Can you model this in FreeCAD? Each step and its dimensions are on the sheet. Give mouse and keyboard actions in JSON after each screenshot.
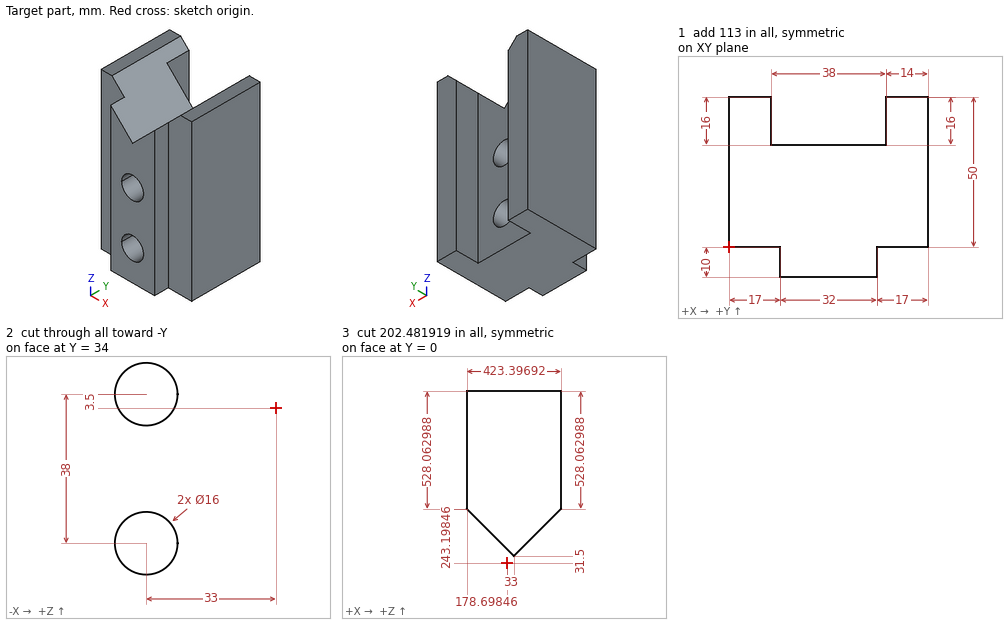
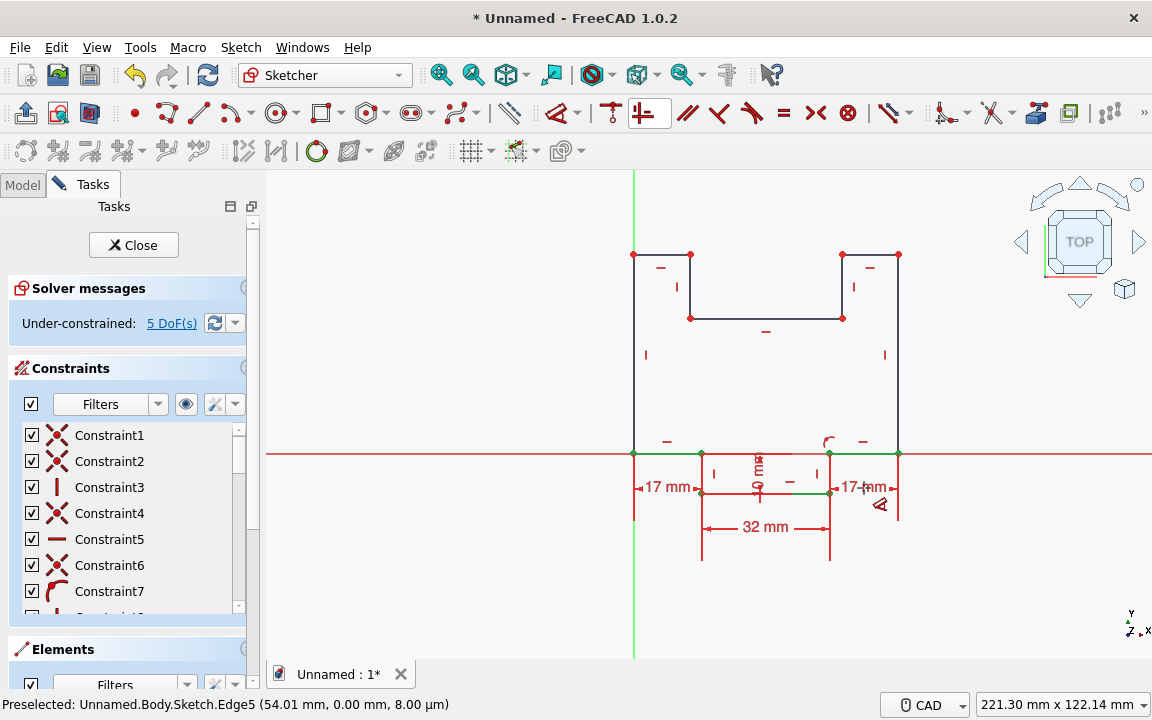
{"action": "left_click", "coordinate": [898, 394]}
{"action": "left_click", "coordinate": [932, 354]}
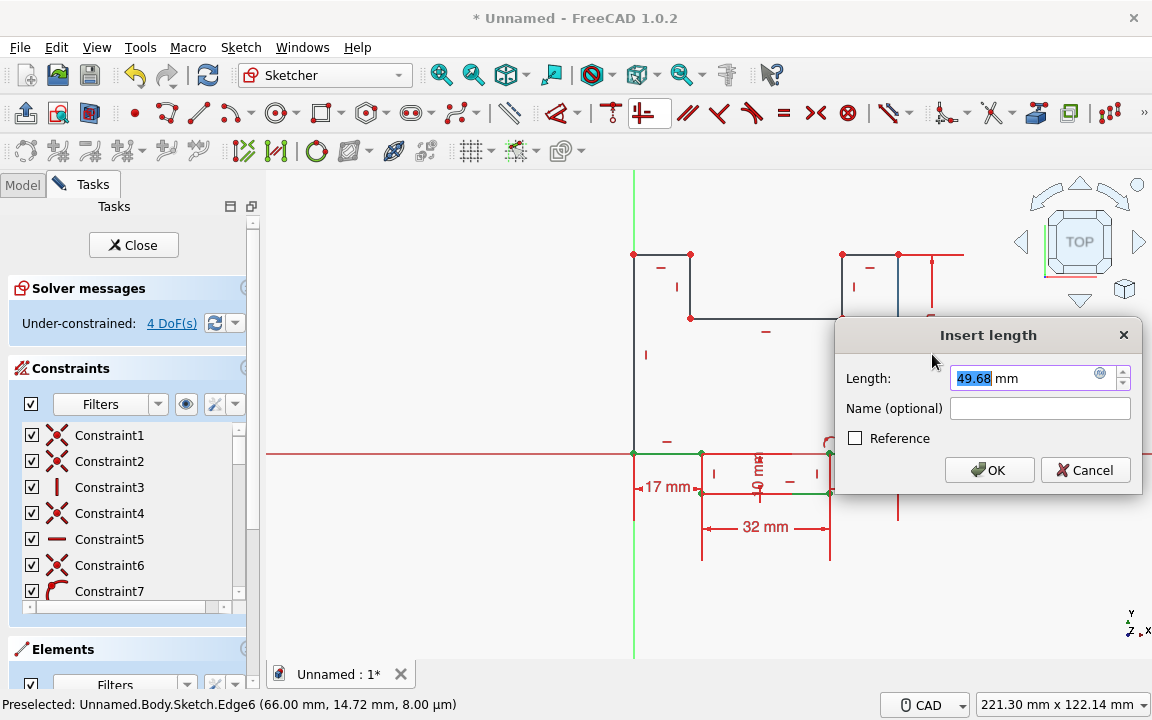
{"action": "type", "text": "50"}
{"action": "key", "text": "Return"}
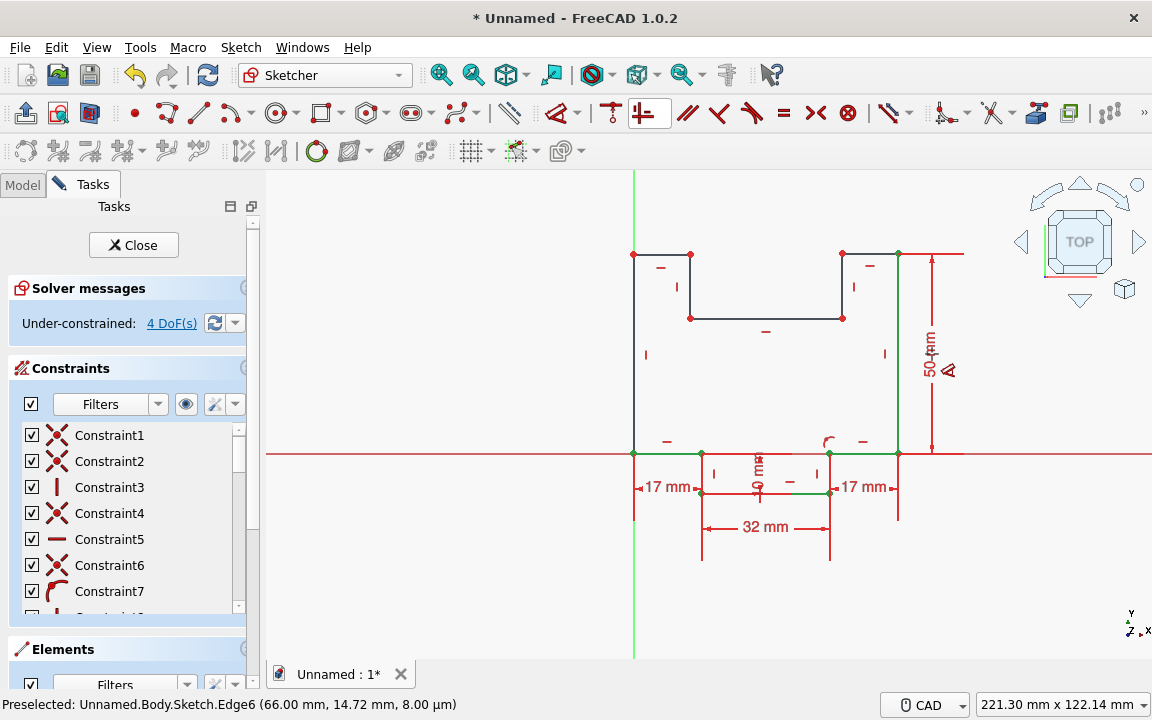
{"action": "left_click", "coordinate": [881, 254]}
{"action": "left_click", "coordinate": [870, 220]}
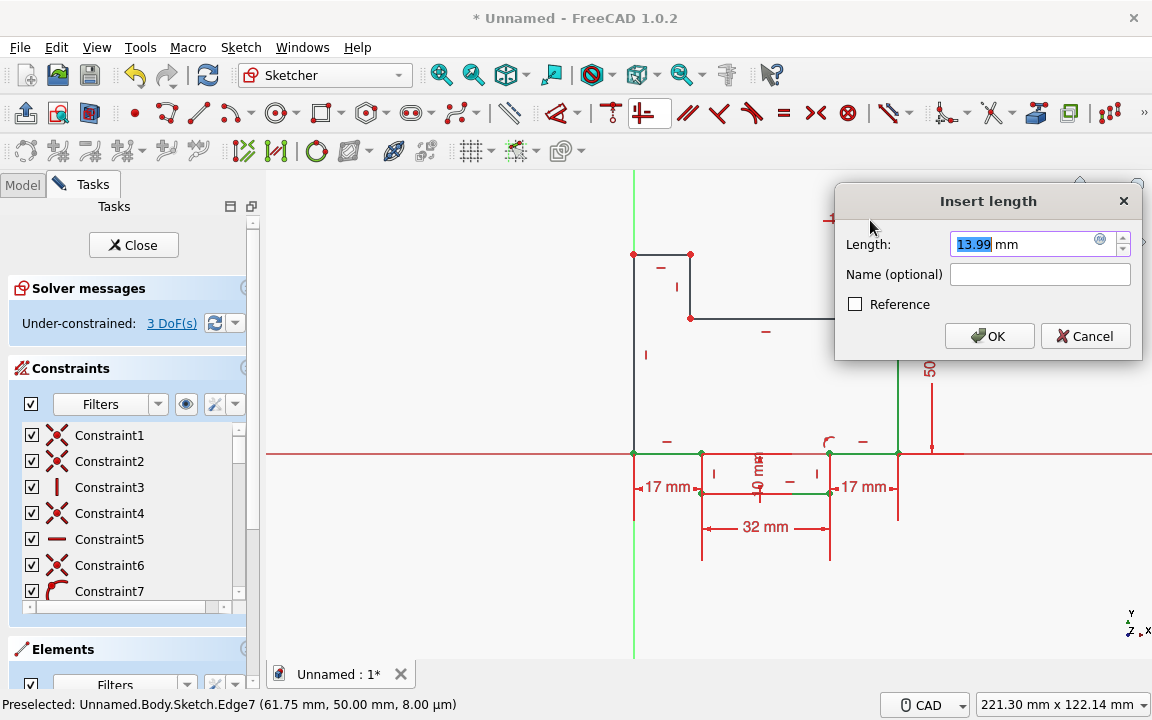
{"action": "type", "text": "14"}
{"action": "key", "text": "Return"}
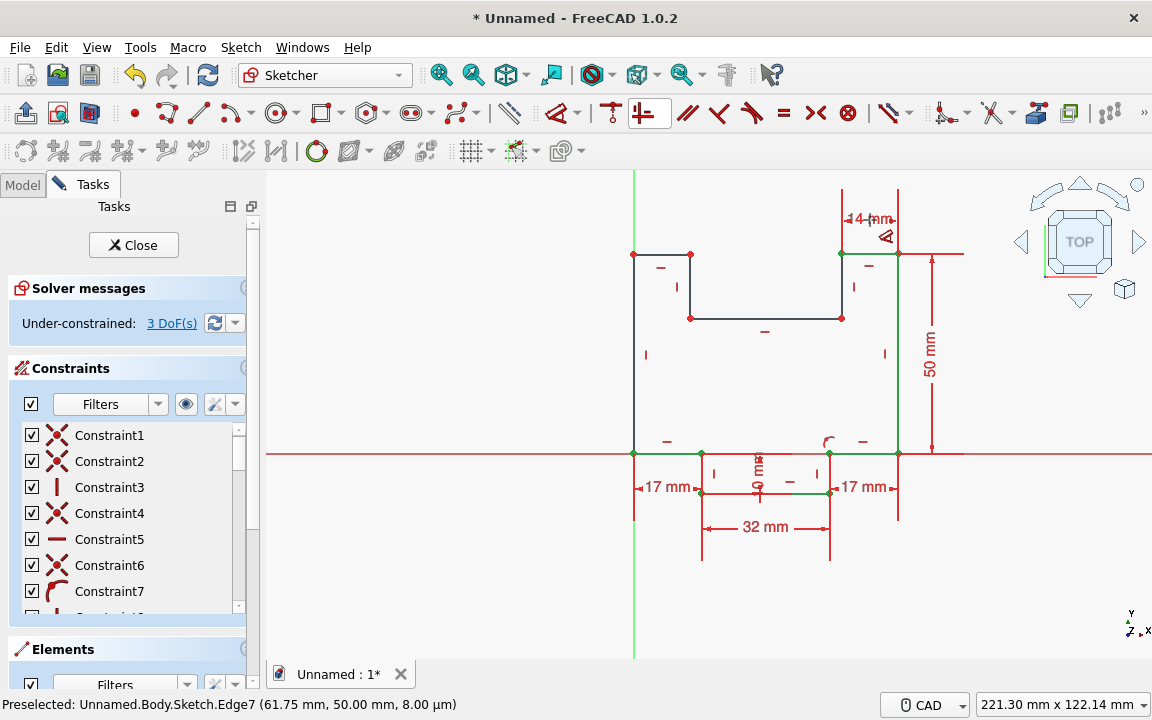
{"action": "left_click", "coordinate": [842, 273]}
{"action": "left_click", "coordinate": [876, 286]}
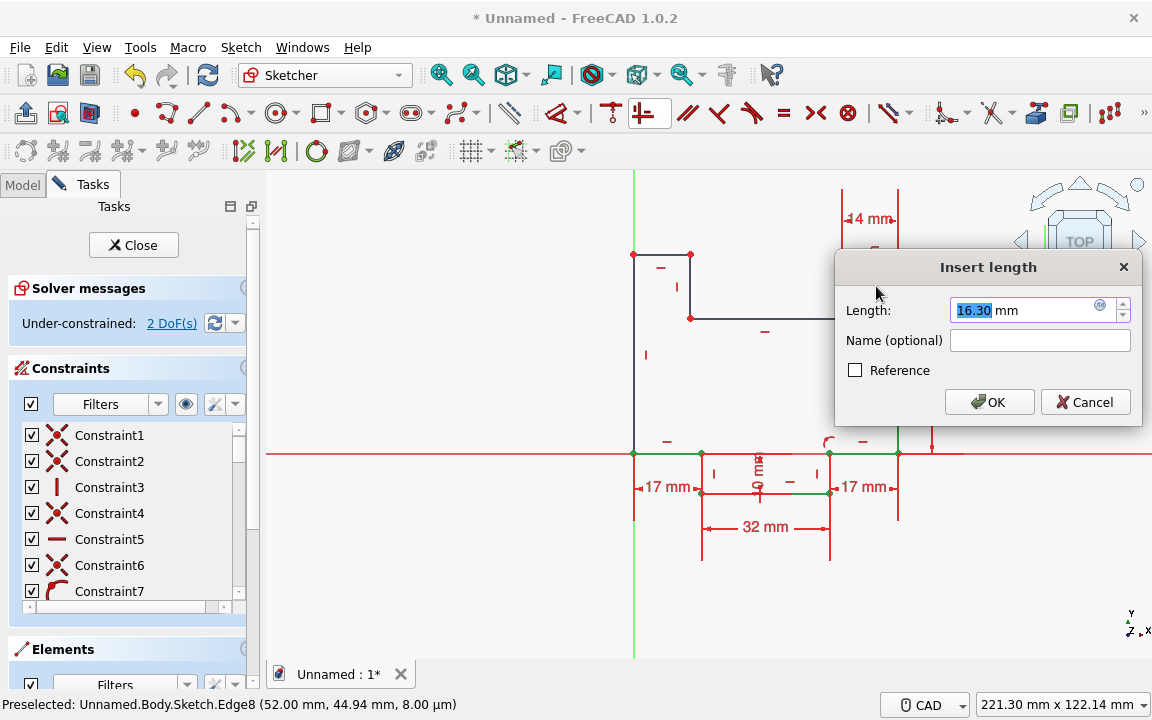
{"action": "type", "text": "16"}
{"action": "key", "text": "Return"}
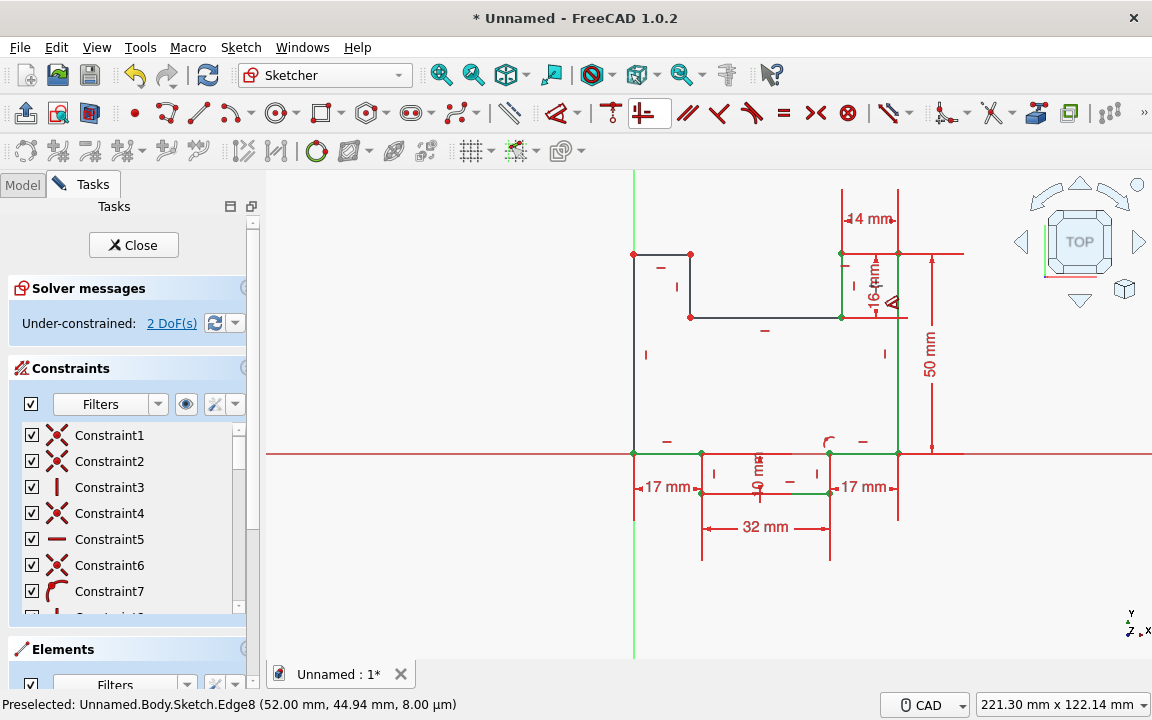
{"action": "left_click", "coordinate": [796, 318]}
{"action": "left_click", "coordinate": [766, 284]}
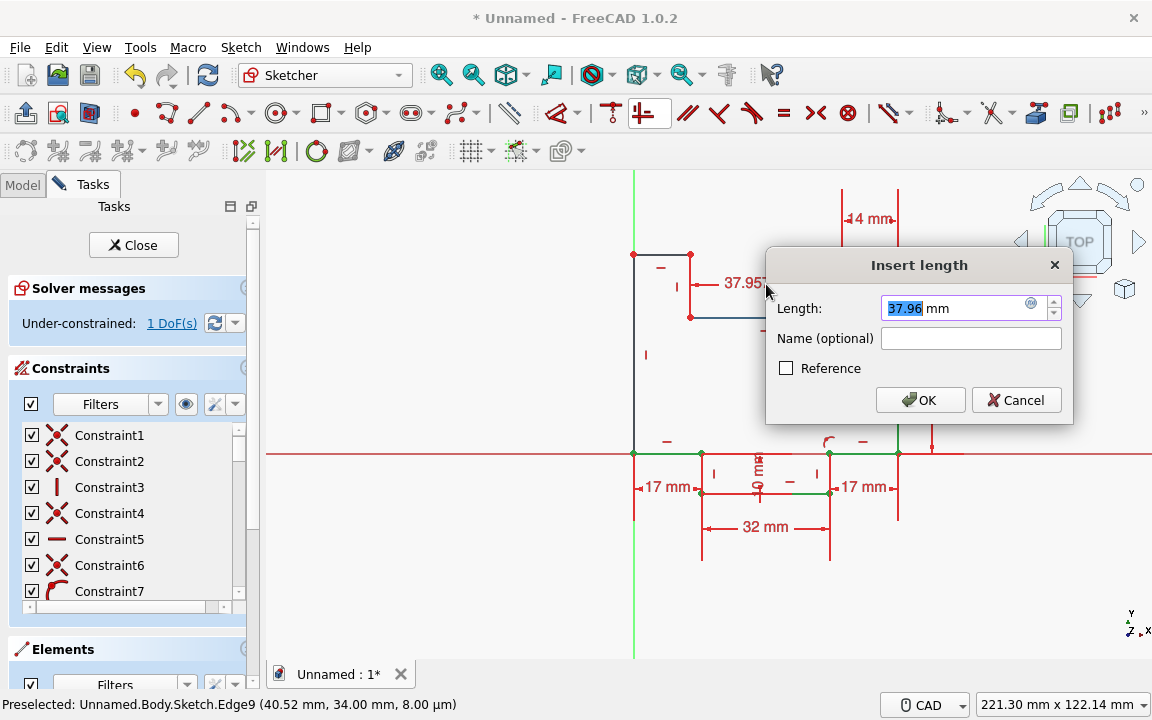
{"action": "type", "text": "38"}
{"action": "key", "text": "Return"}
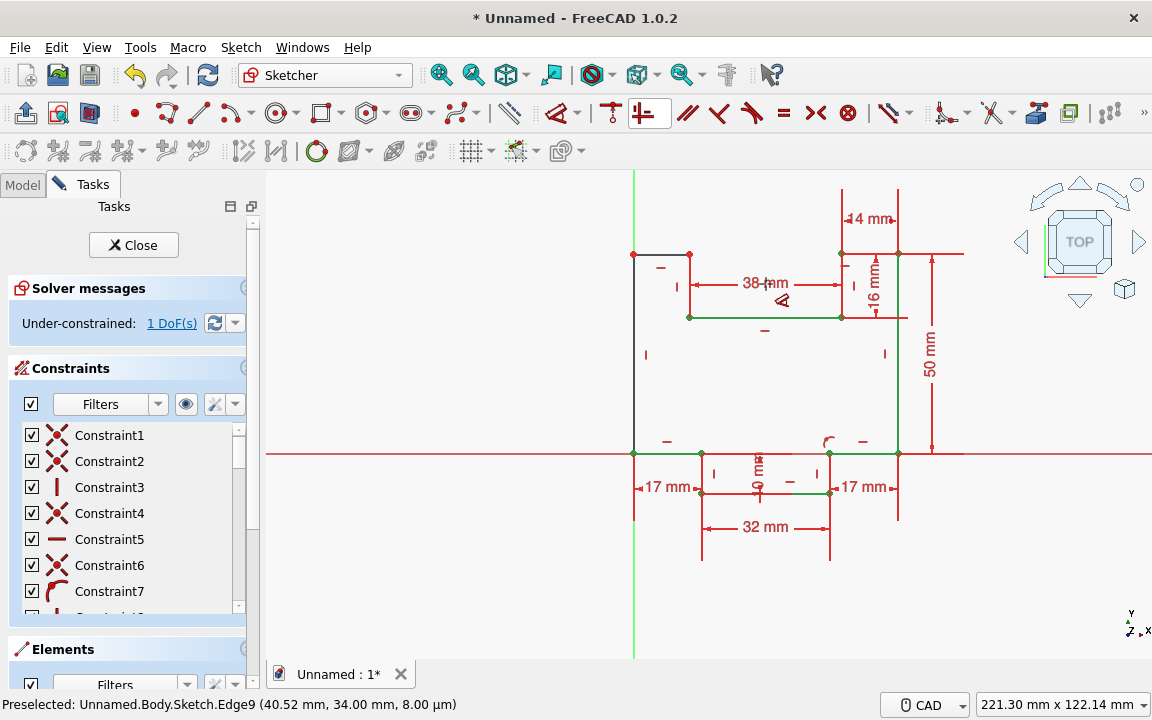
{"action": "left_click", "coordinate": [690, 299]}
{"action": "left_click", "coordinate": [656, 286]}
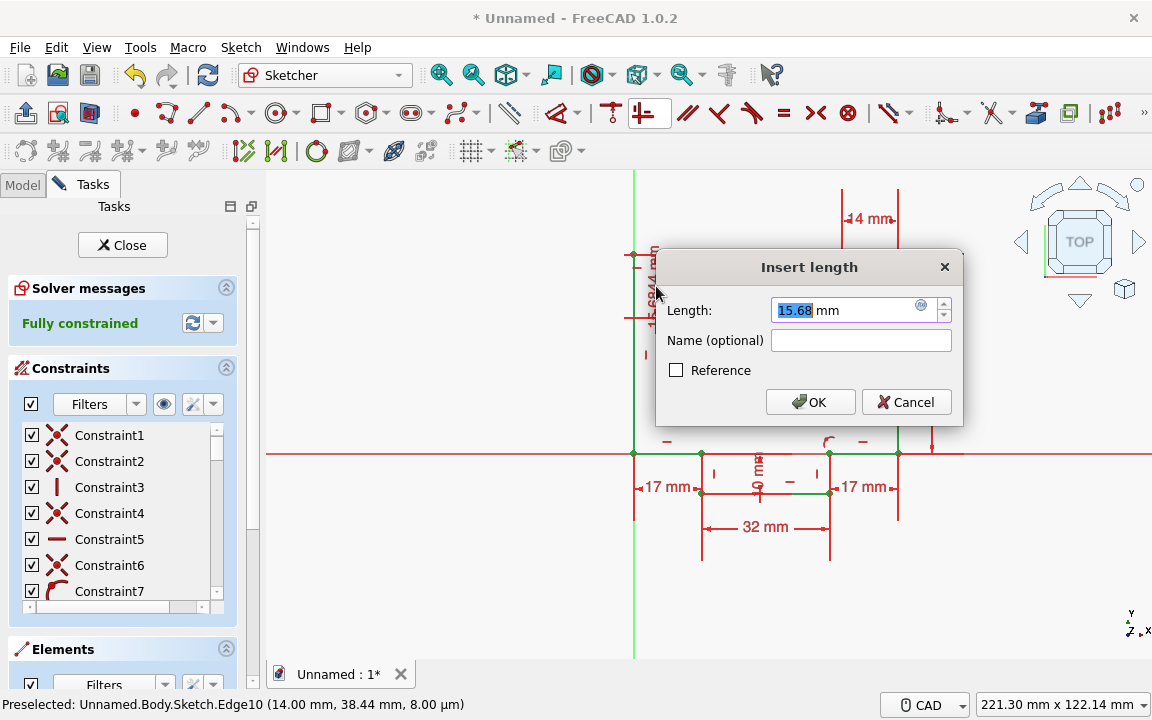
{"action": "type", "text": "16"}
{"action": "key", "text": "Return"}
{"action": "key", "text": "Escape"}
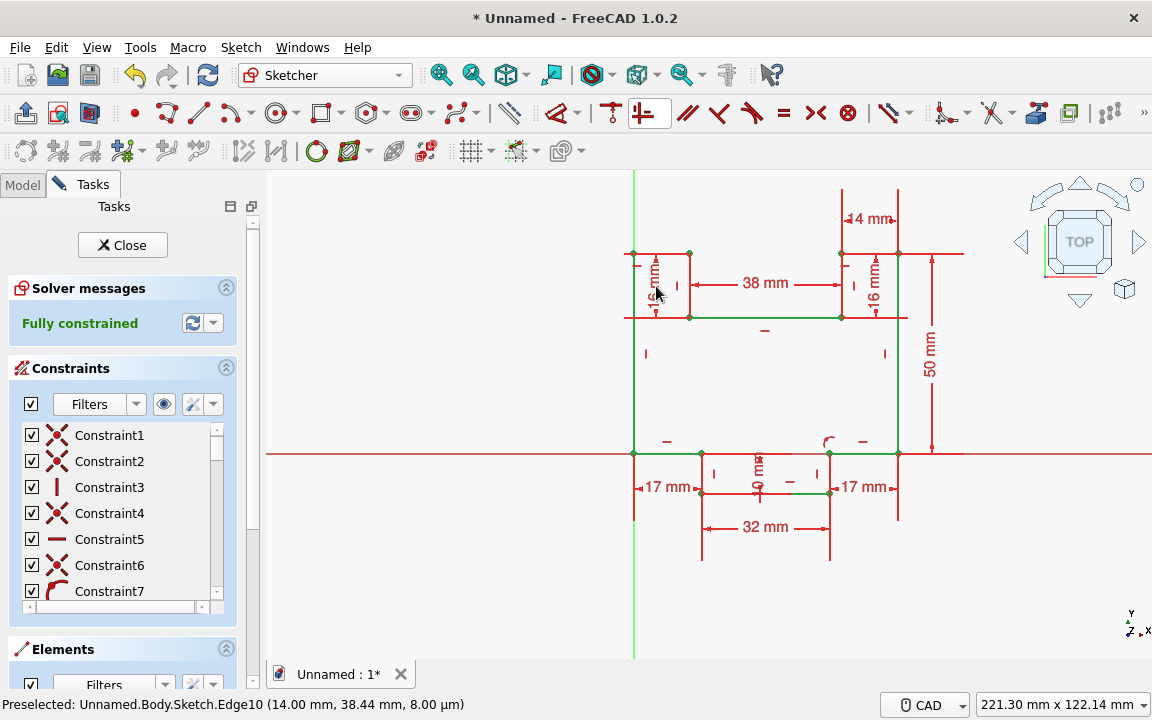
{"action": "left_click", "coordinate": [123, 245]}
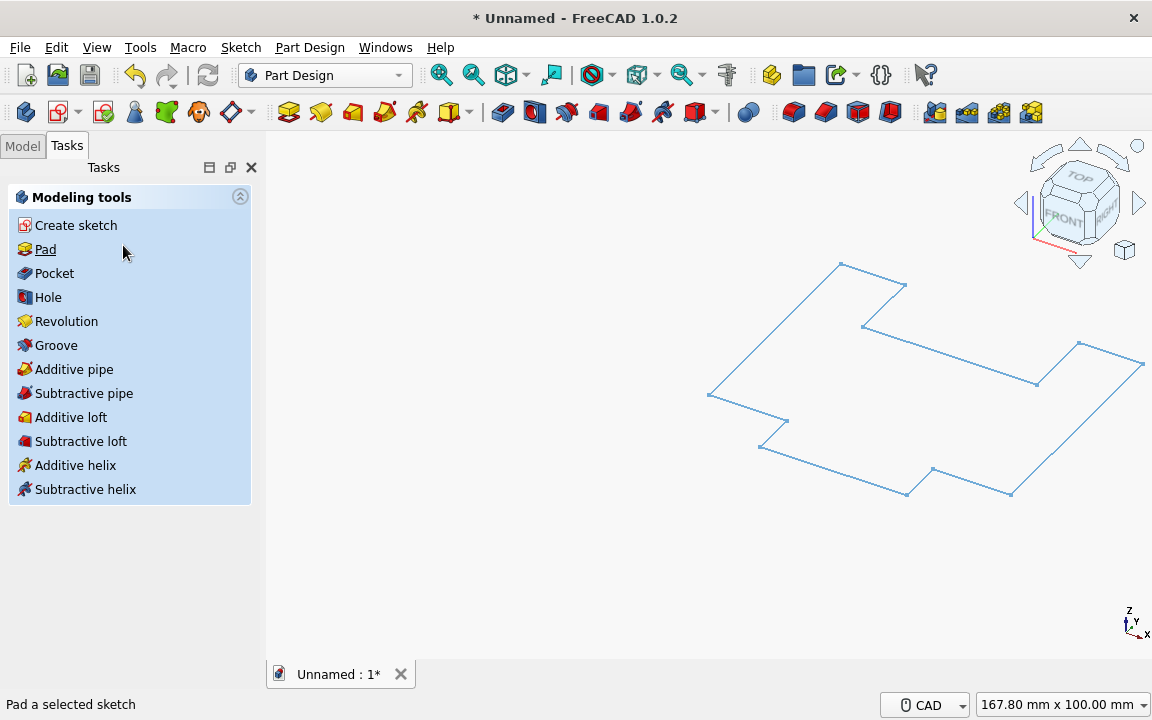
{"action": "left_click", "coordinate": [290, 112]}